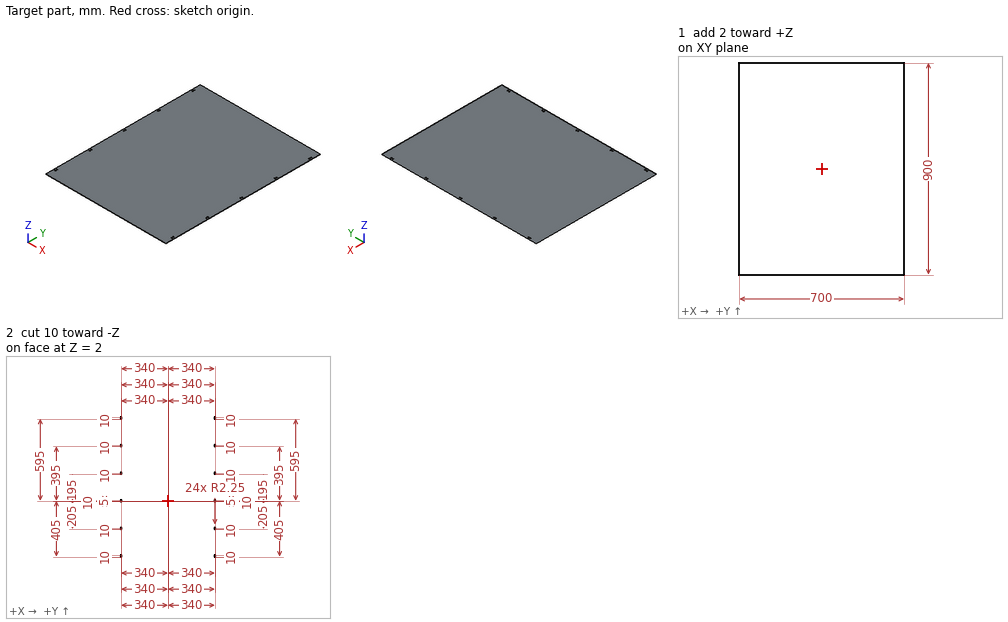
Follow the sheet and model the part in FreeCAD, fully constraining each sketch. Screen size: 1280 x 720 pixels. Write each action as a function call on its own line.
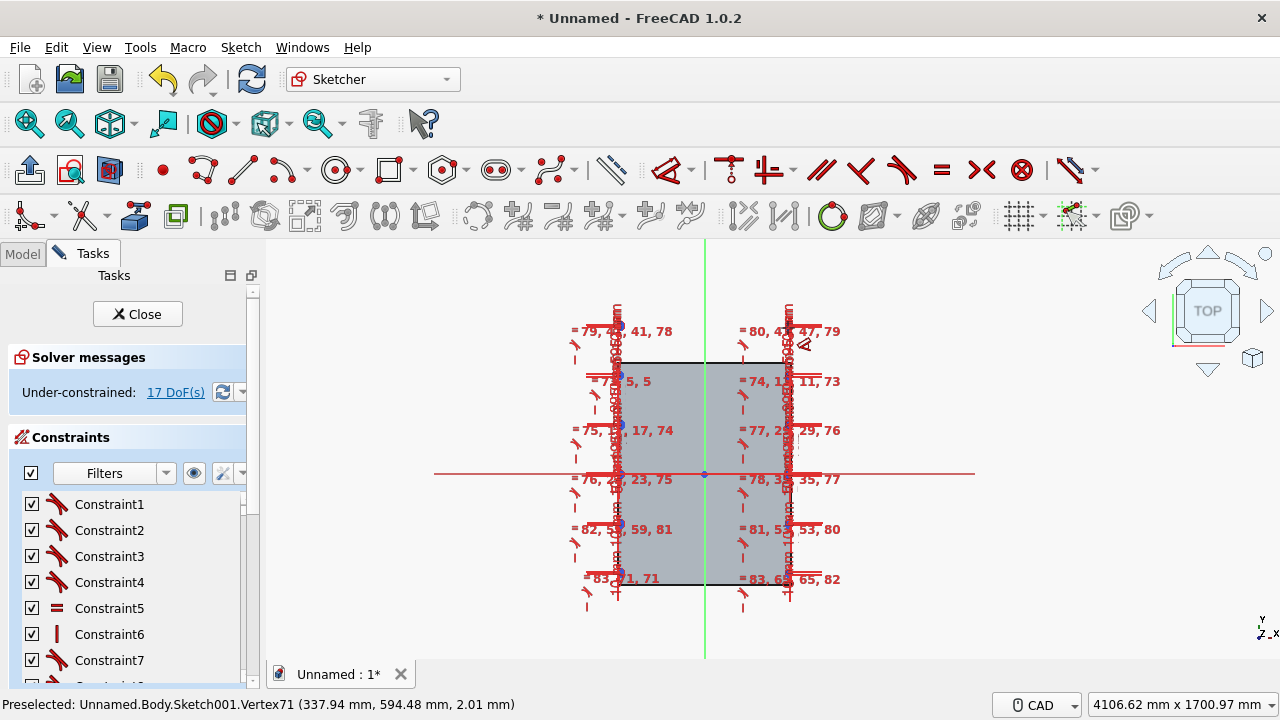
scroll(789, 525, up, 14)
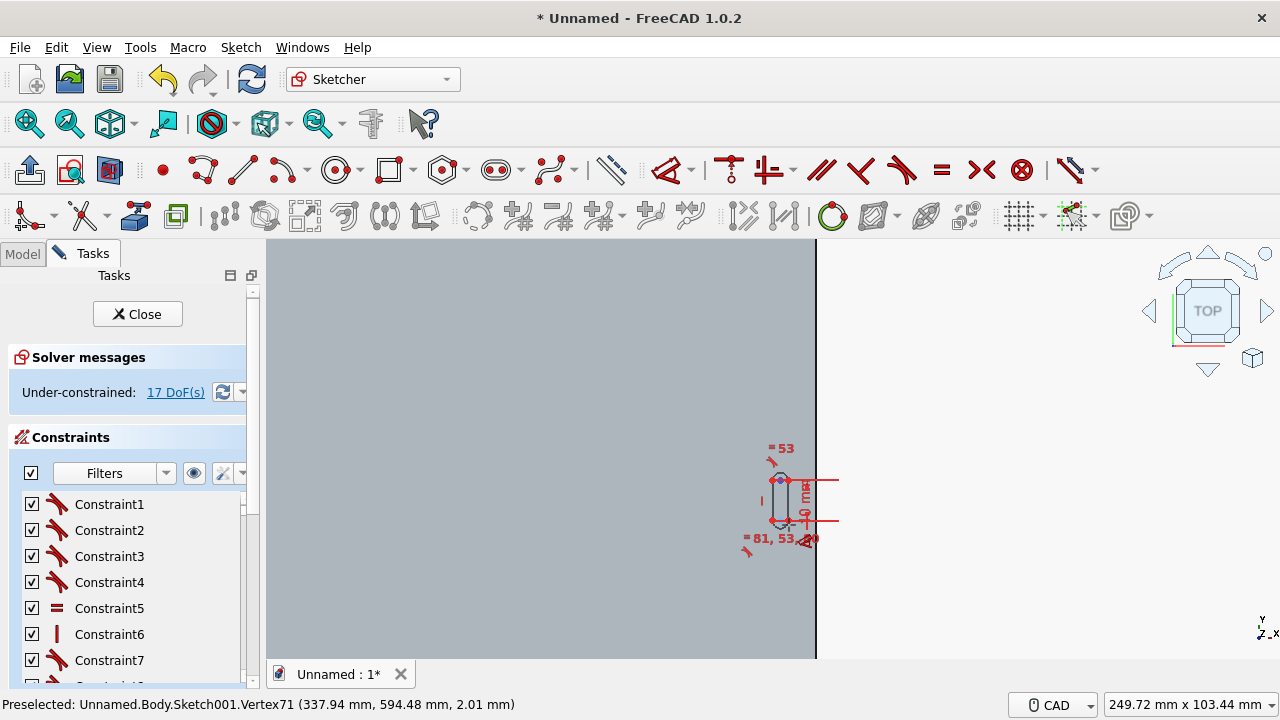
click(773, 521)
click(807, 394)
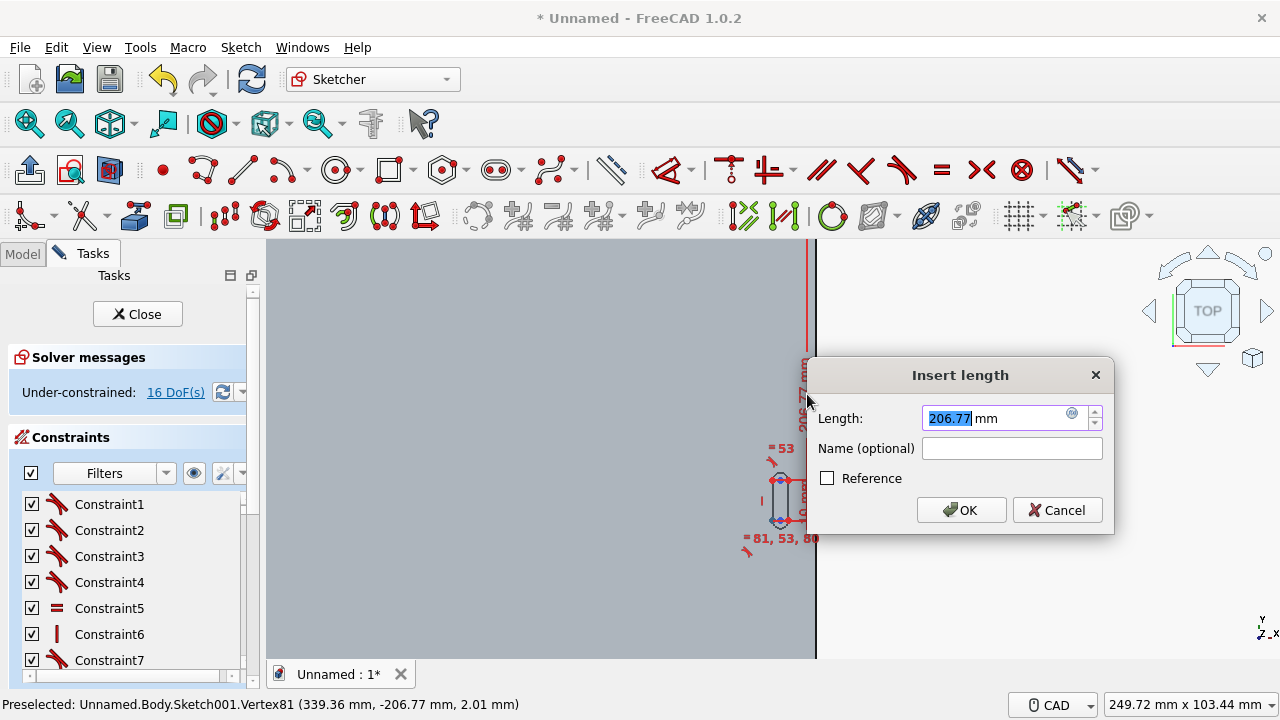
text(205)
key(Return)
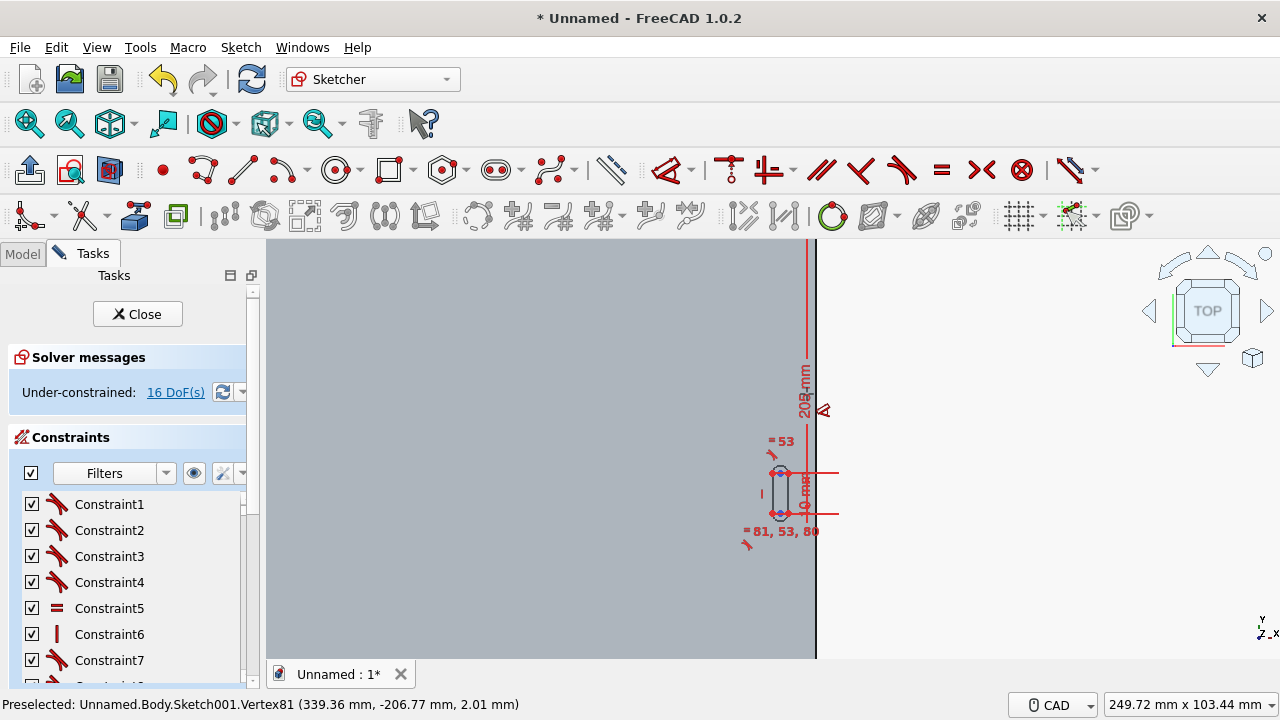
scroll(789, 525, down, 14)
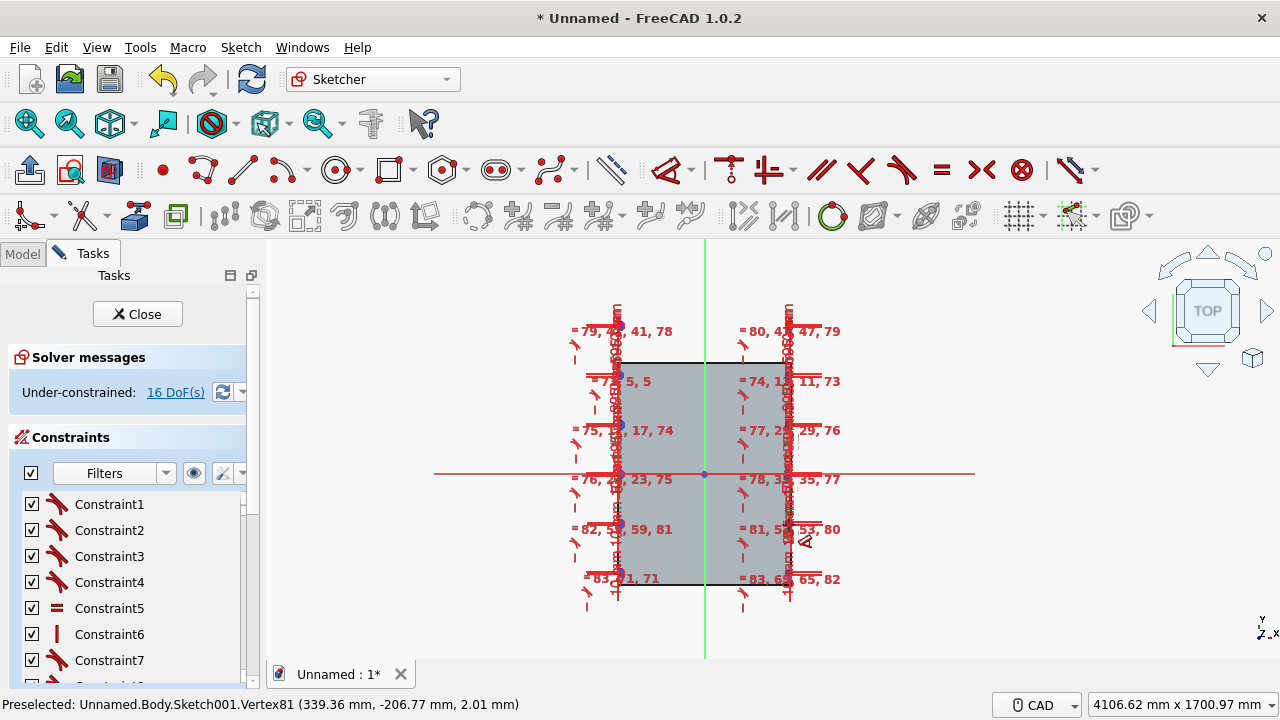
scroll(621, 525, up, 14)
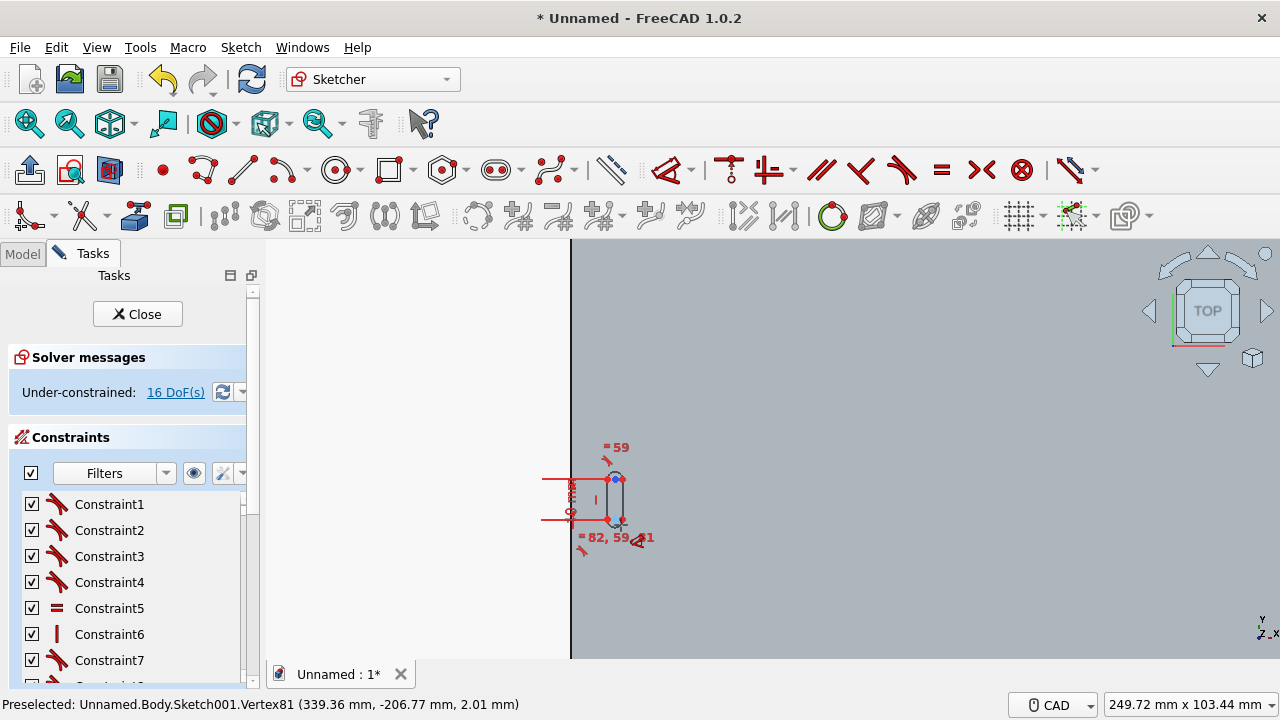
click(607, 520)
click(573, 393)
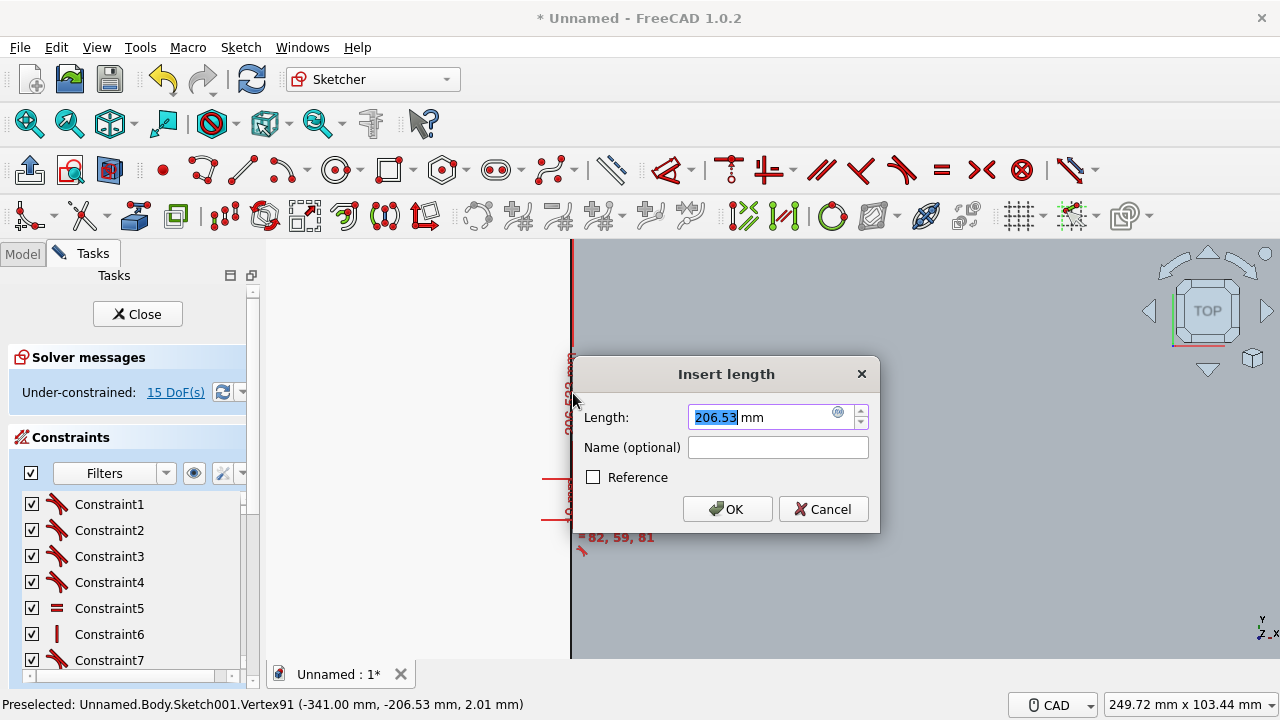
text(205)
key(Return)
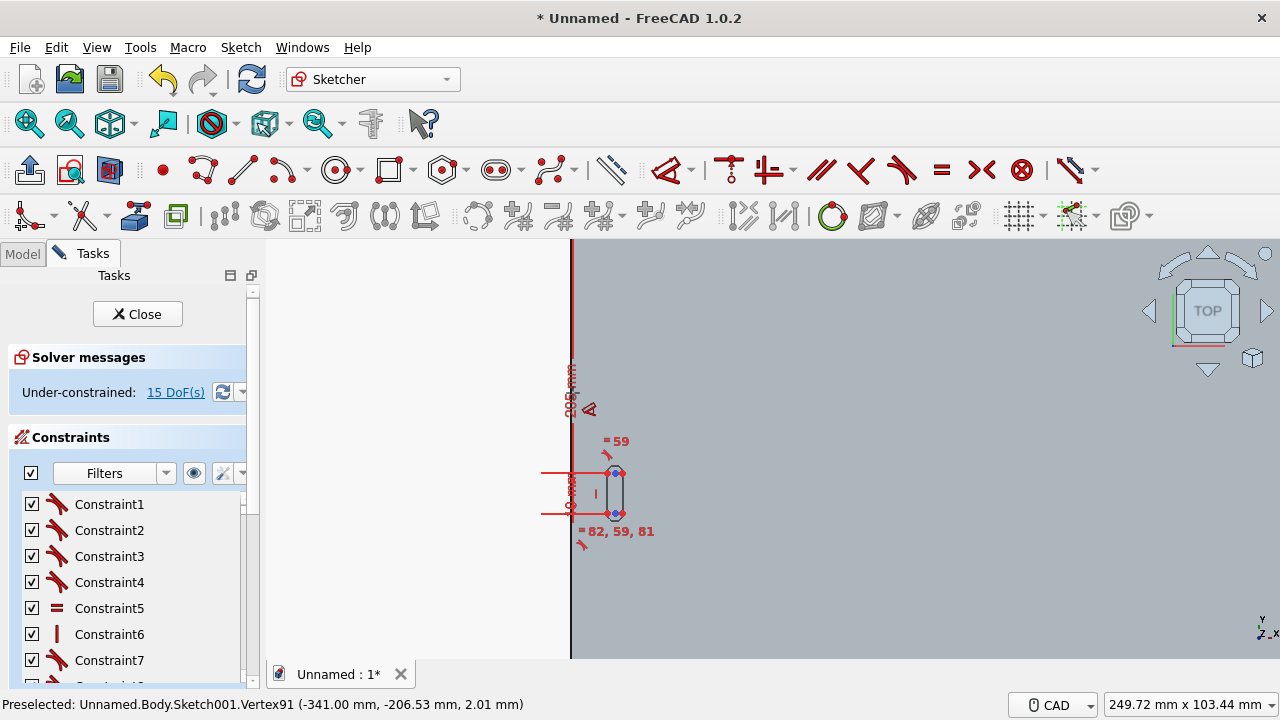
scroll(621, 525, down, 14)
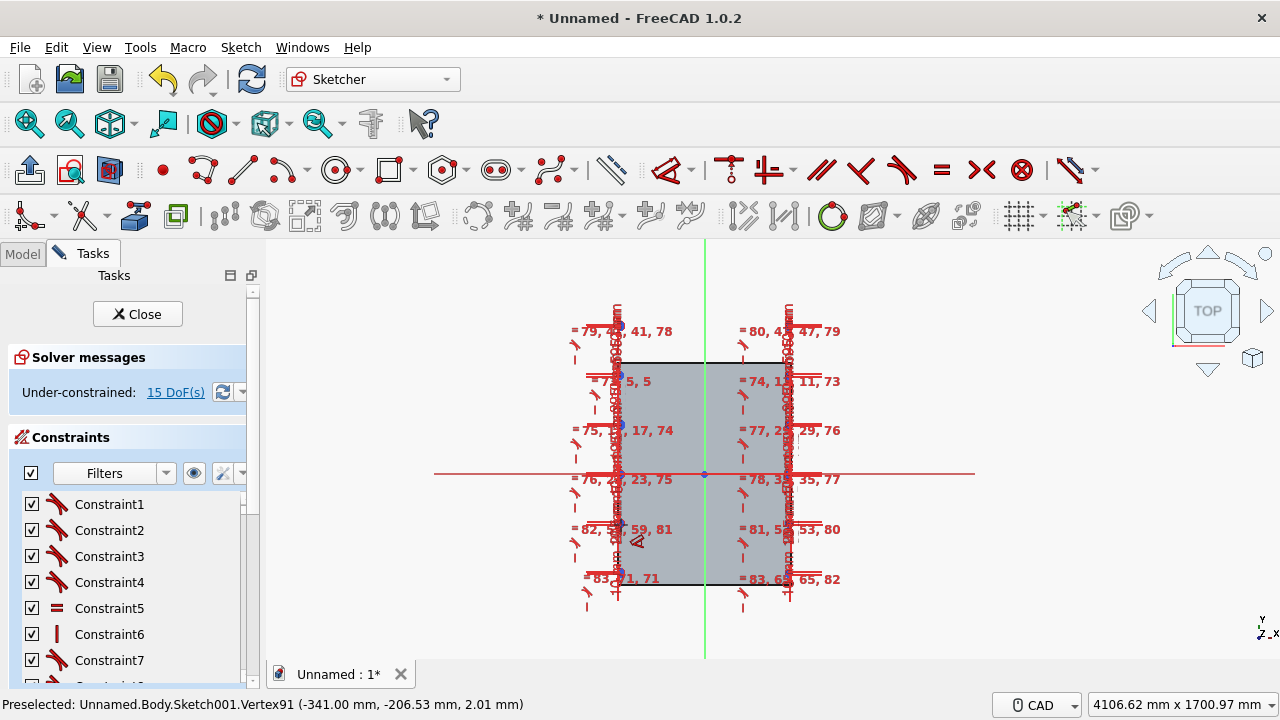
scroll(788, 575, up, 14)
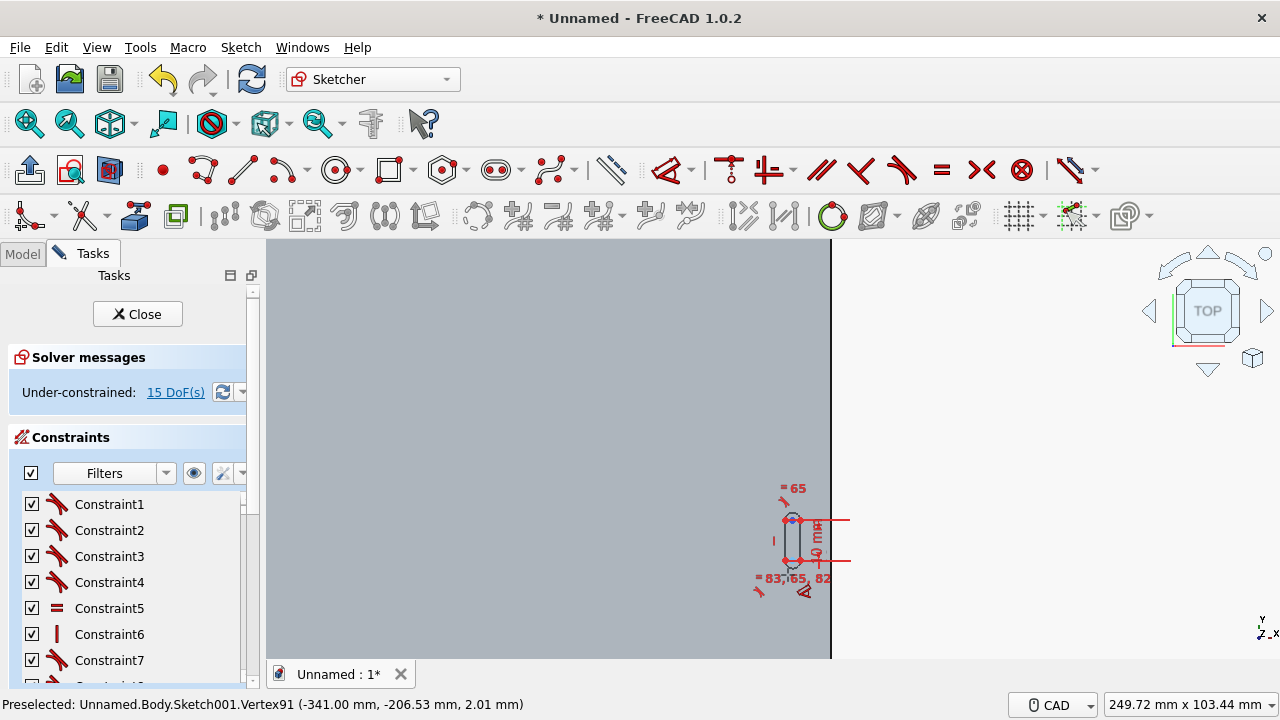
click(785, 561)
click(819, 414)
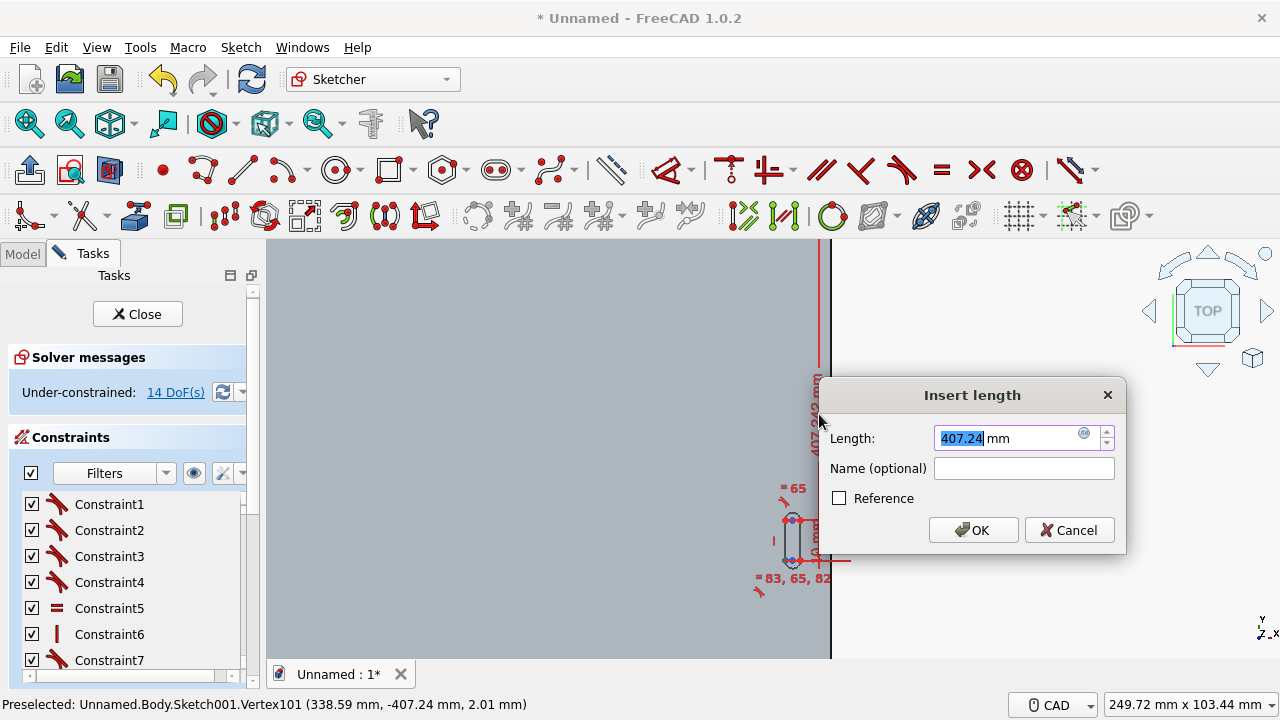
text(405)
key(Return)